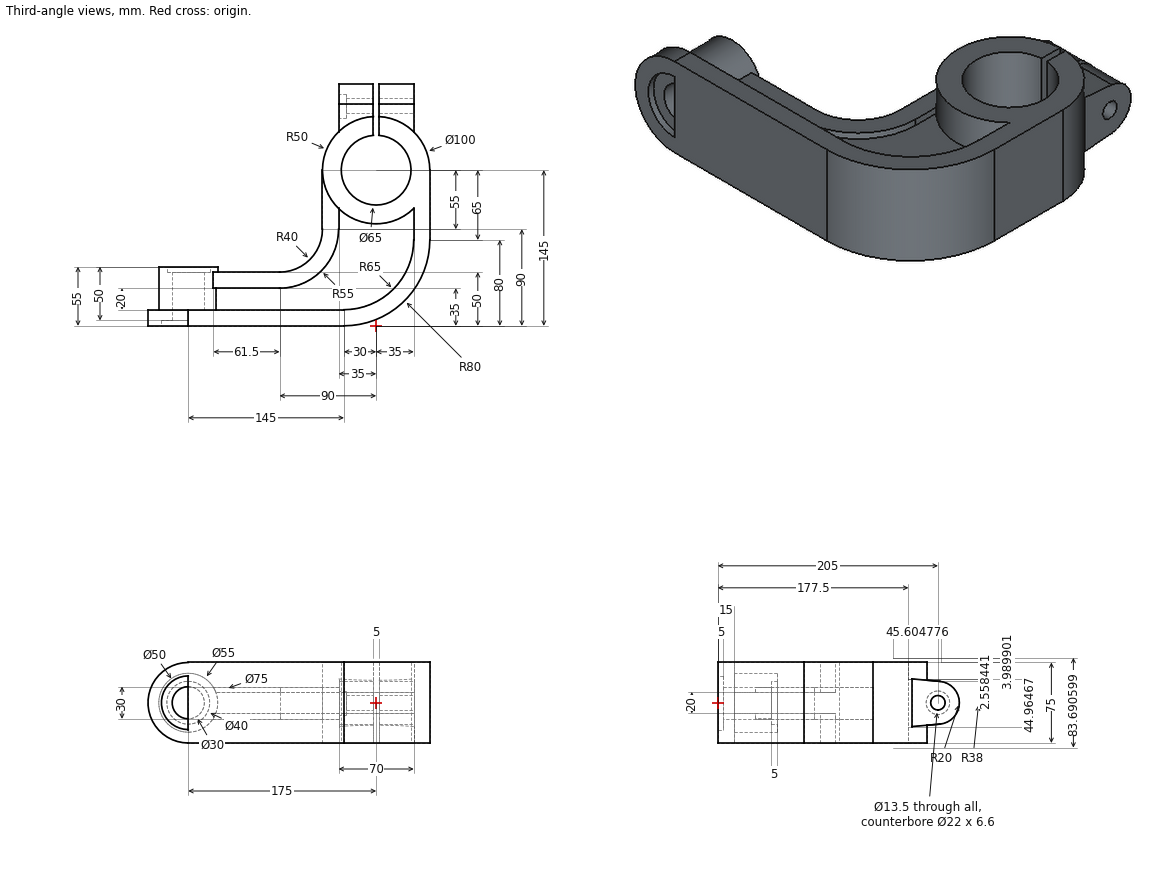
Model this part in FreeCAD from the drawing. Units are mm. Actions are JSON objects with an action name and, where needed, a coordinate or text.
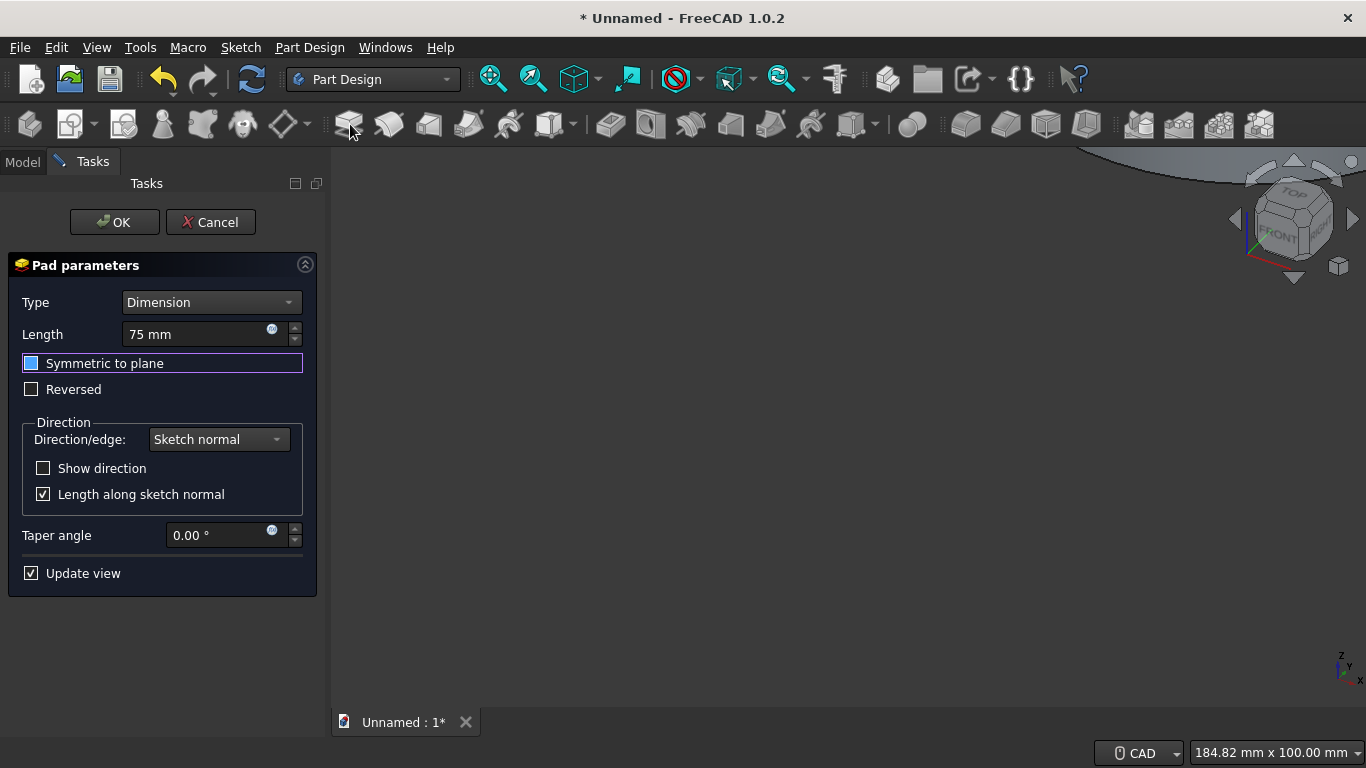
{"action": "left_click", "coordinate": [30, 363]}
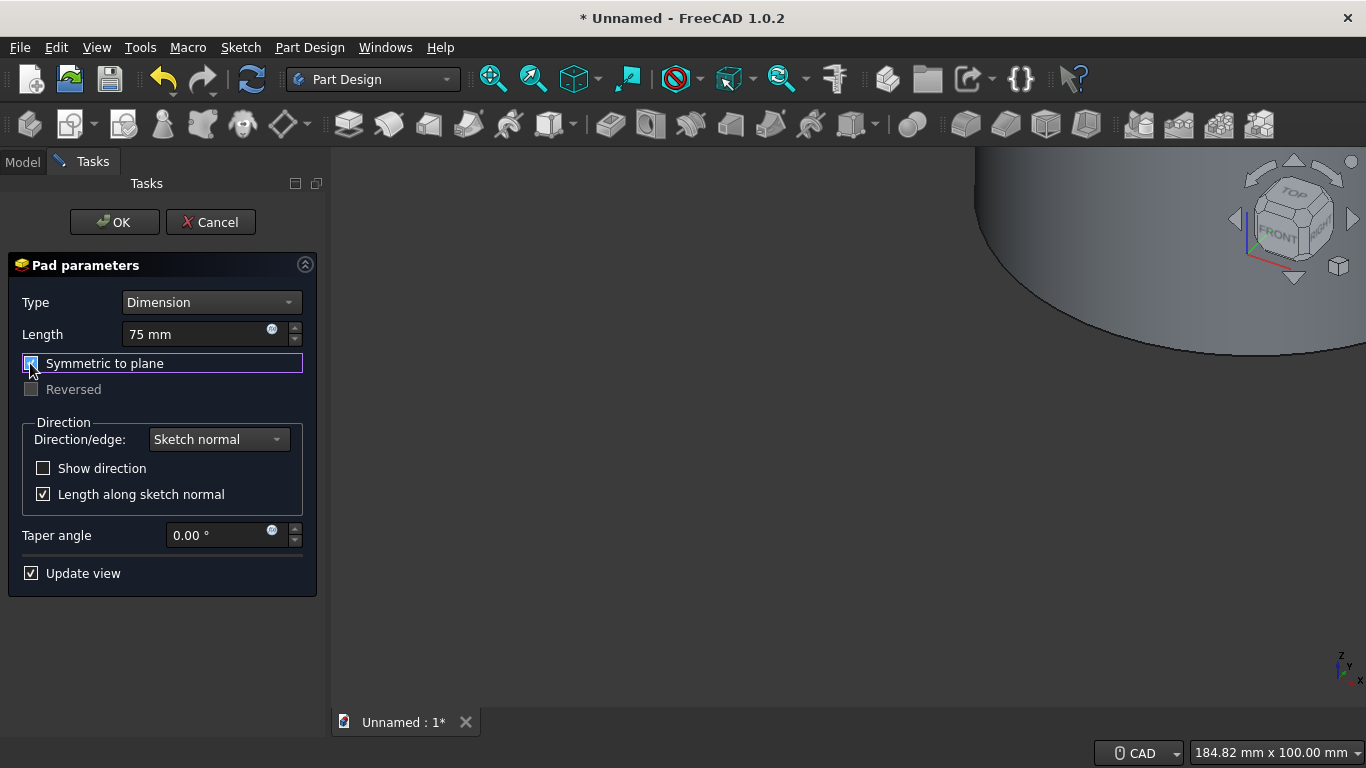
{"action": "left_click", "coordinate": [115, 222]}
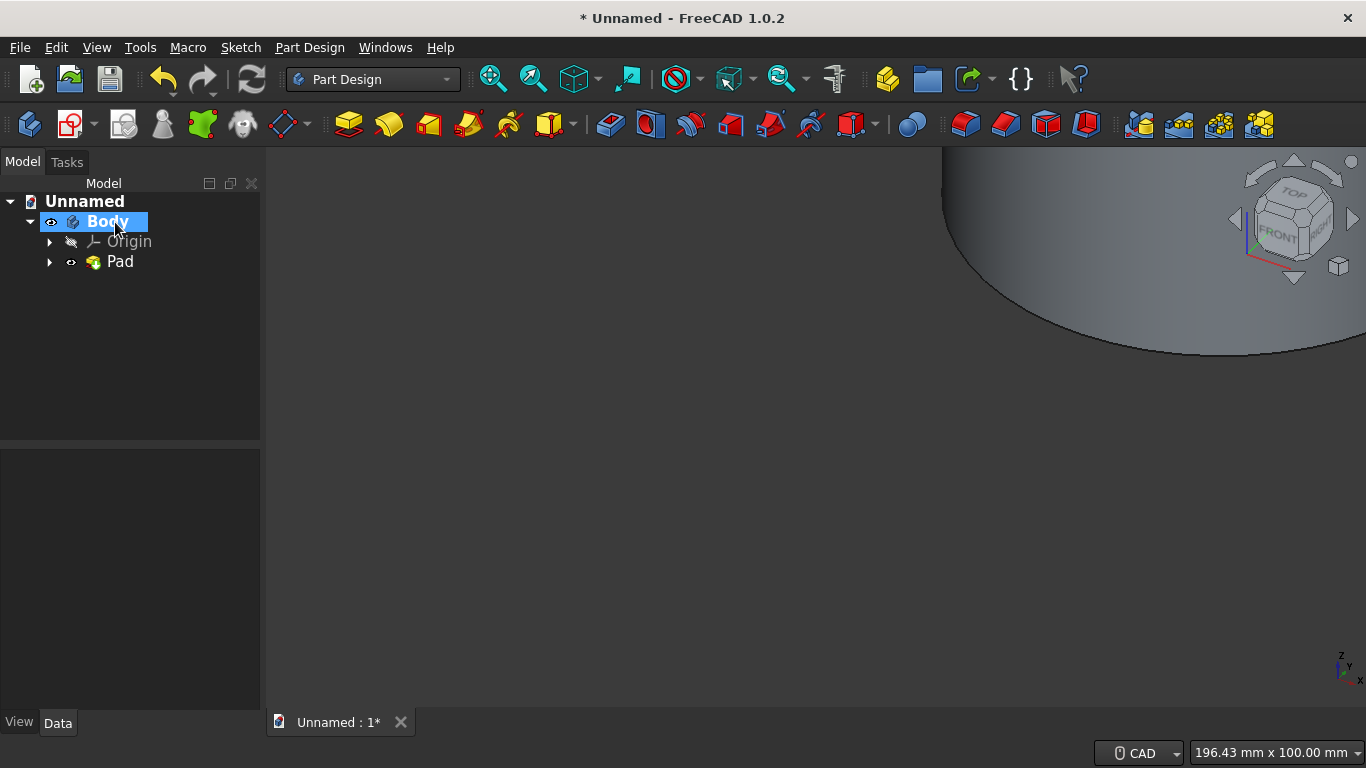
{"action": "left_click", "coordinate": [494, 80]}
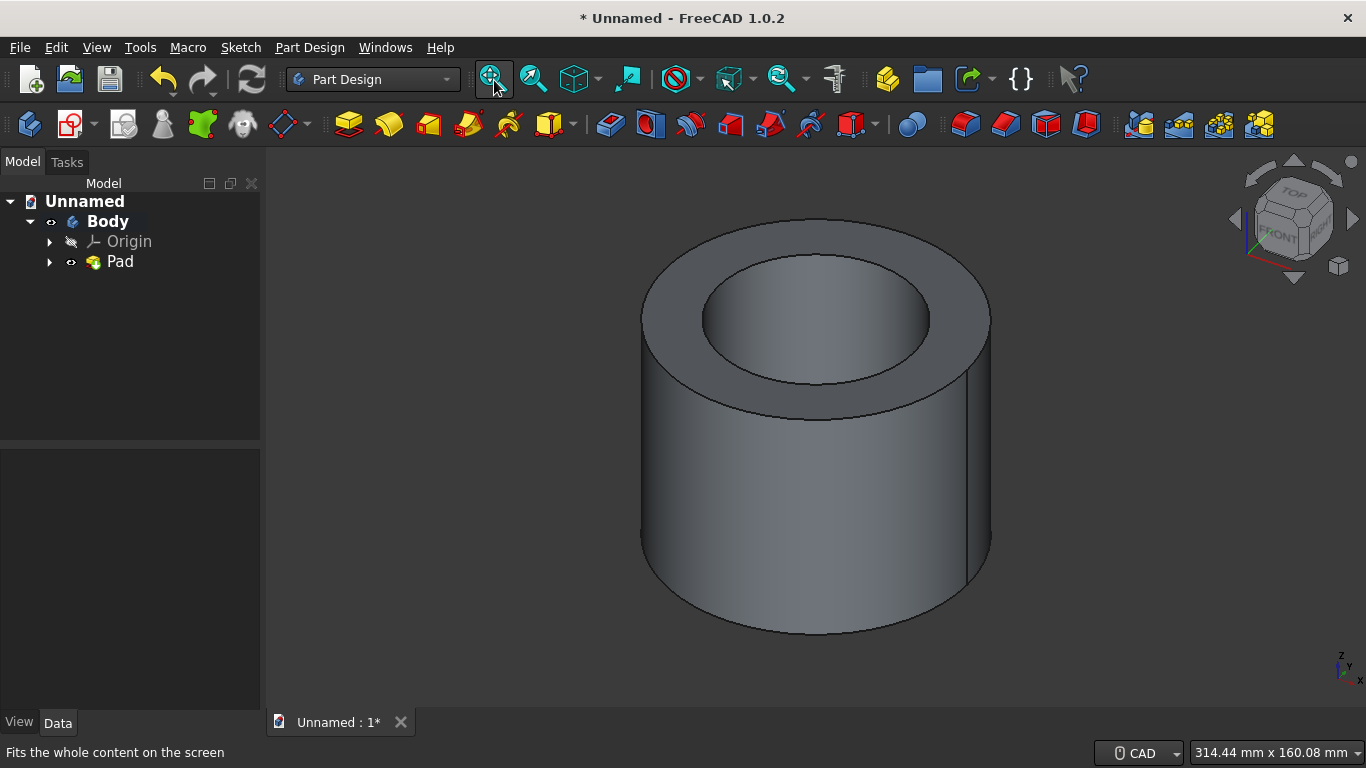
{"action": "left_click", "coordinate": [30, 124]}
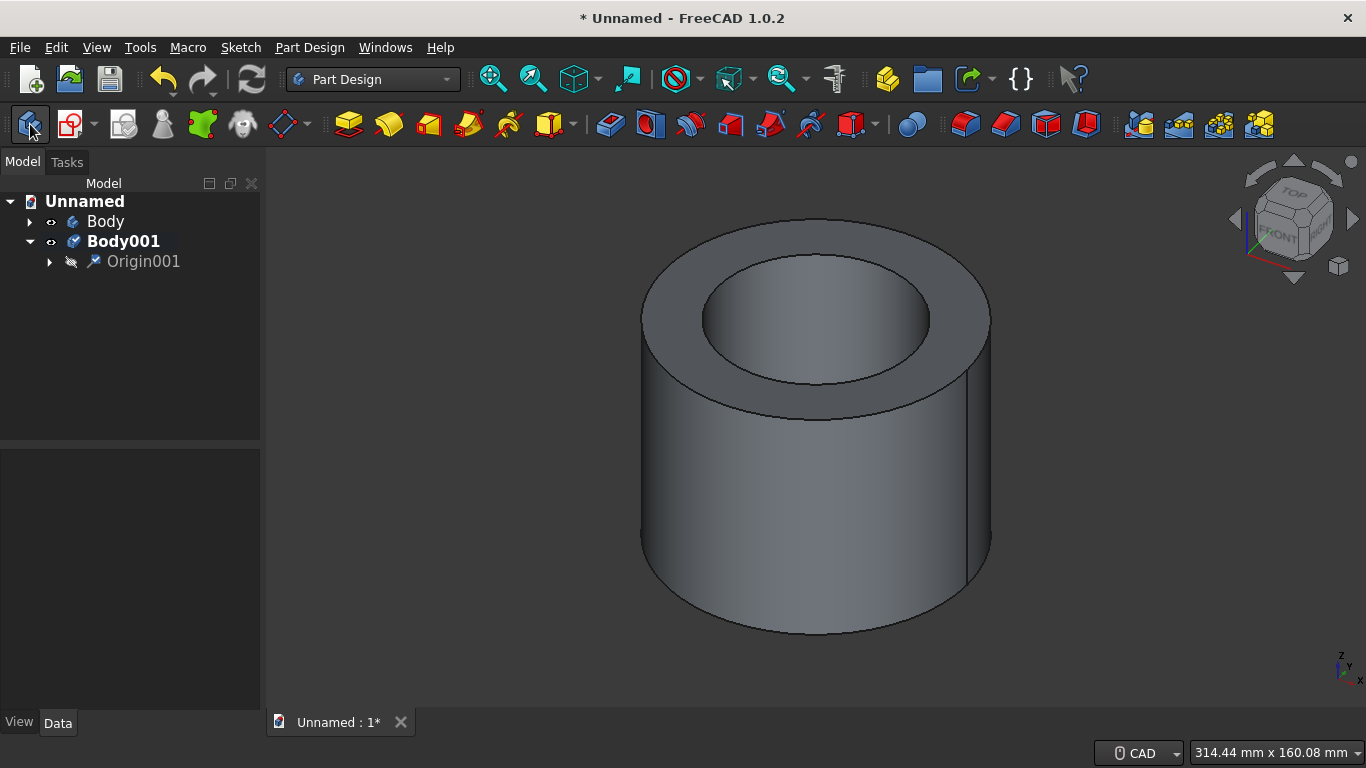
{"action": "left_click", "coordinate": [306, 667]}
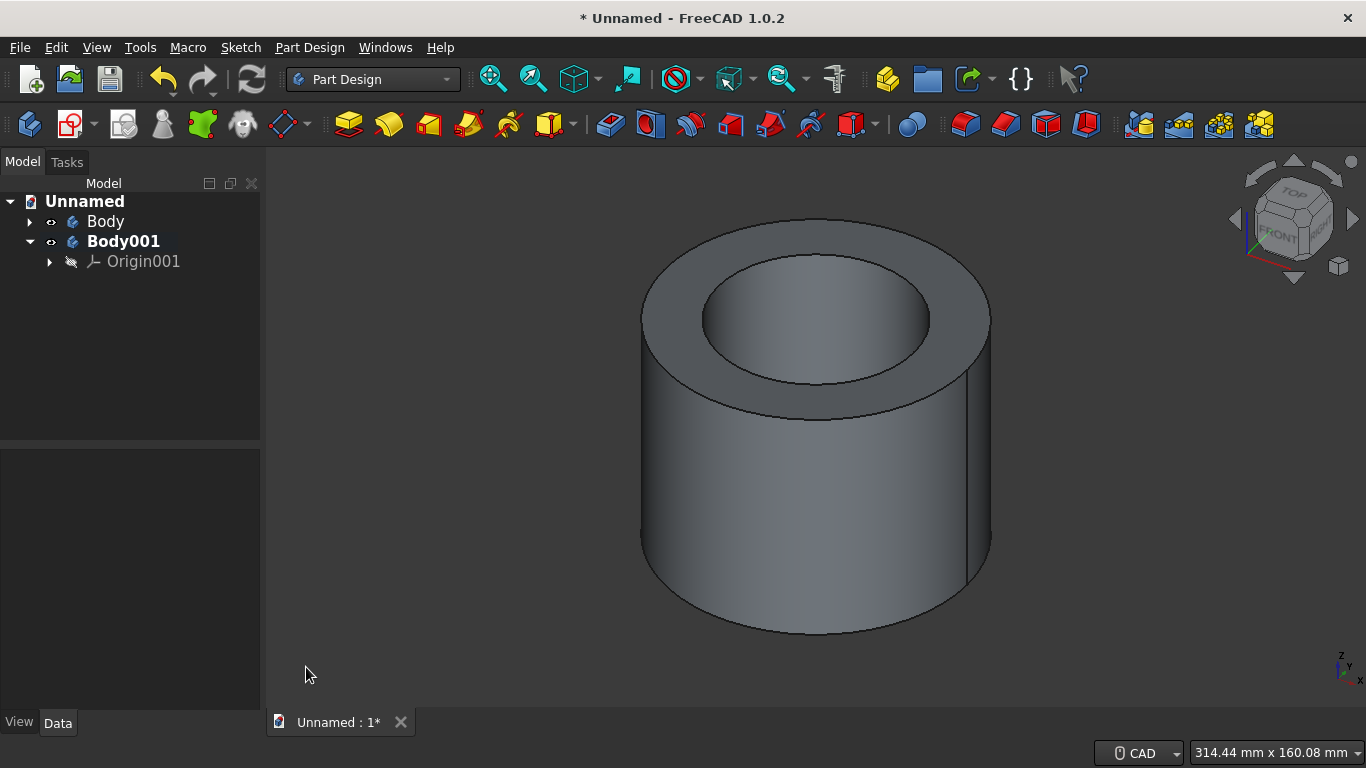
{"action": "left_click", "coordinate": [70, 124]}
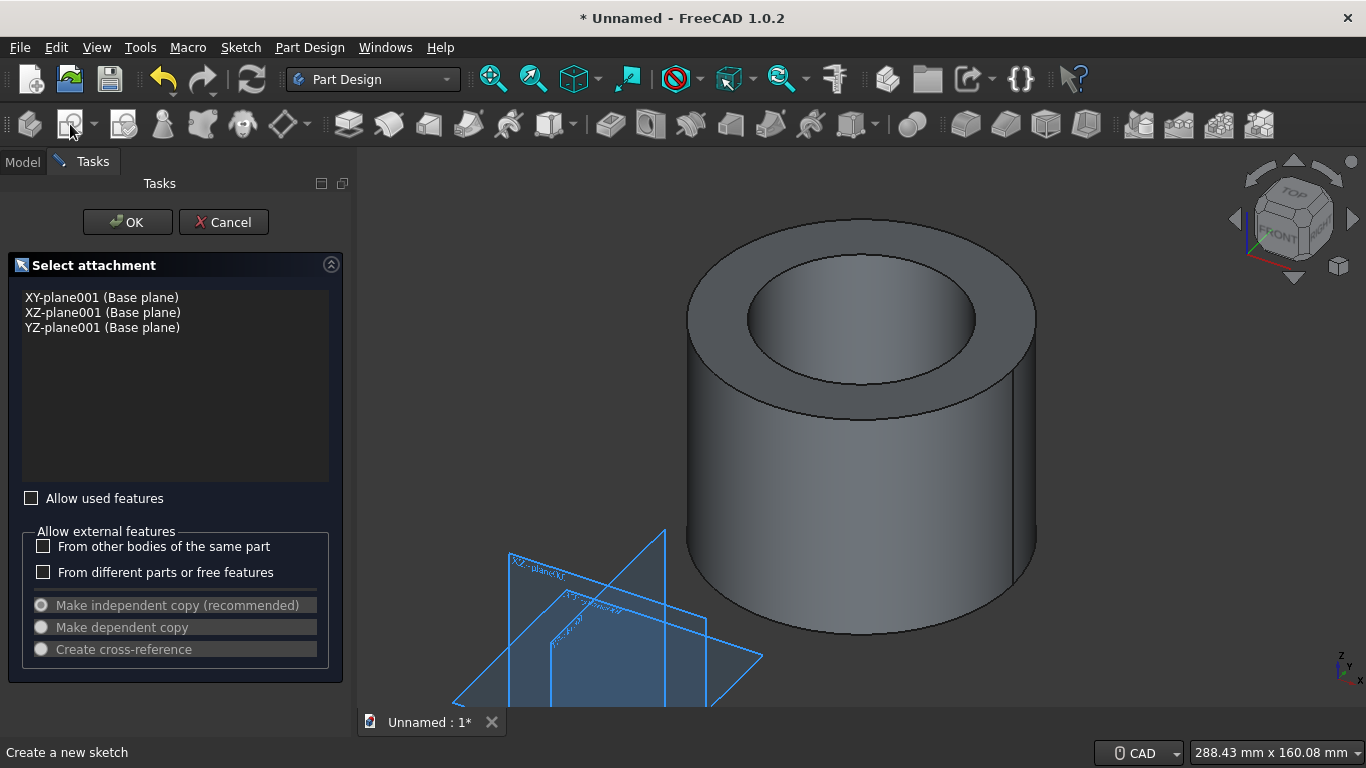
{"action": "left_click", "coordinate": [82, 312]}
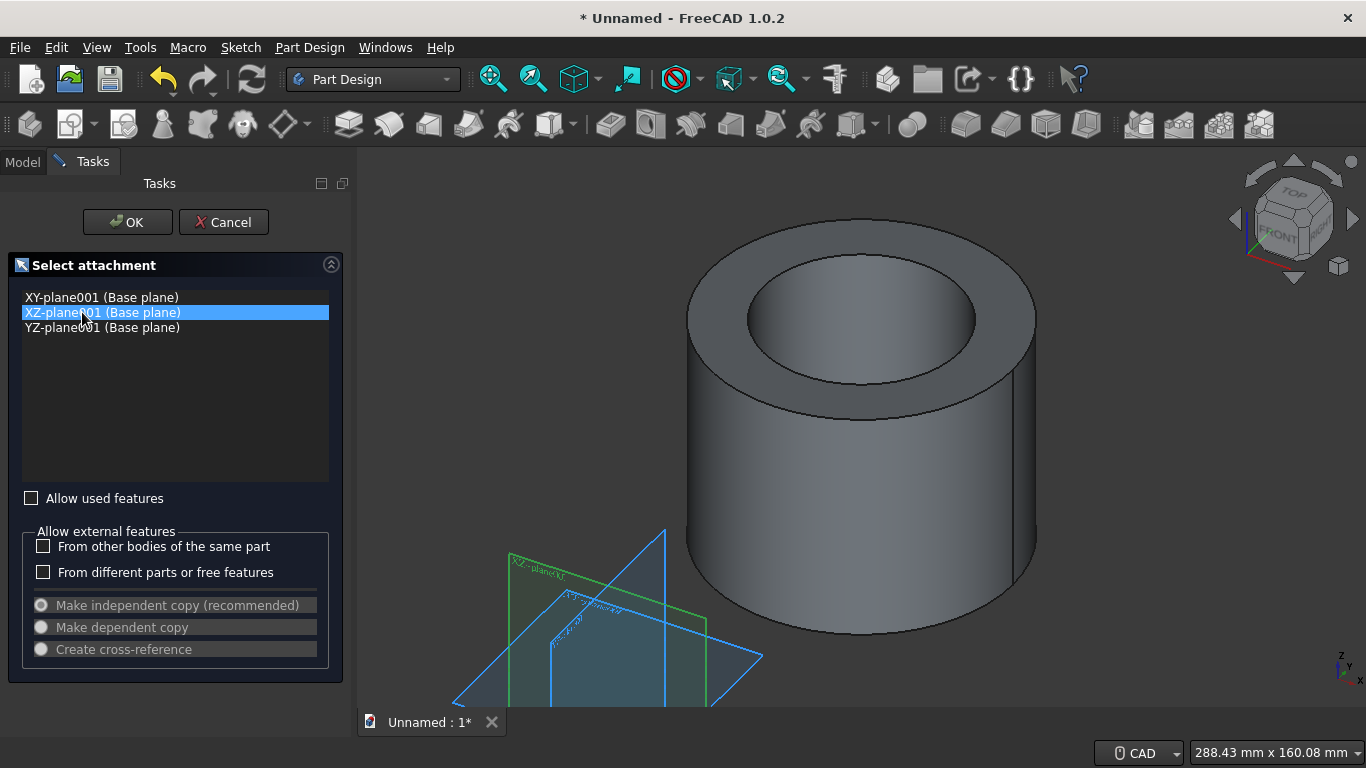
{"action": "left_click", "coordinate": [128, 222]}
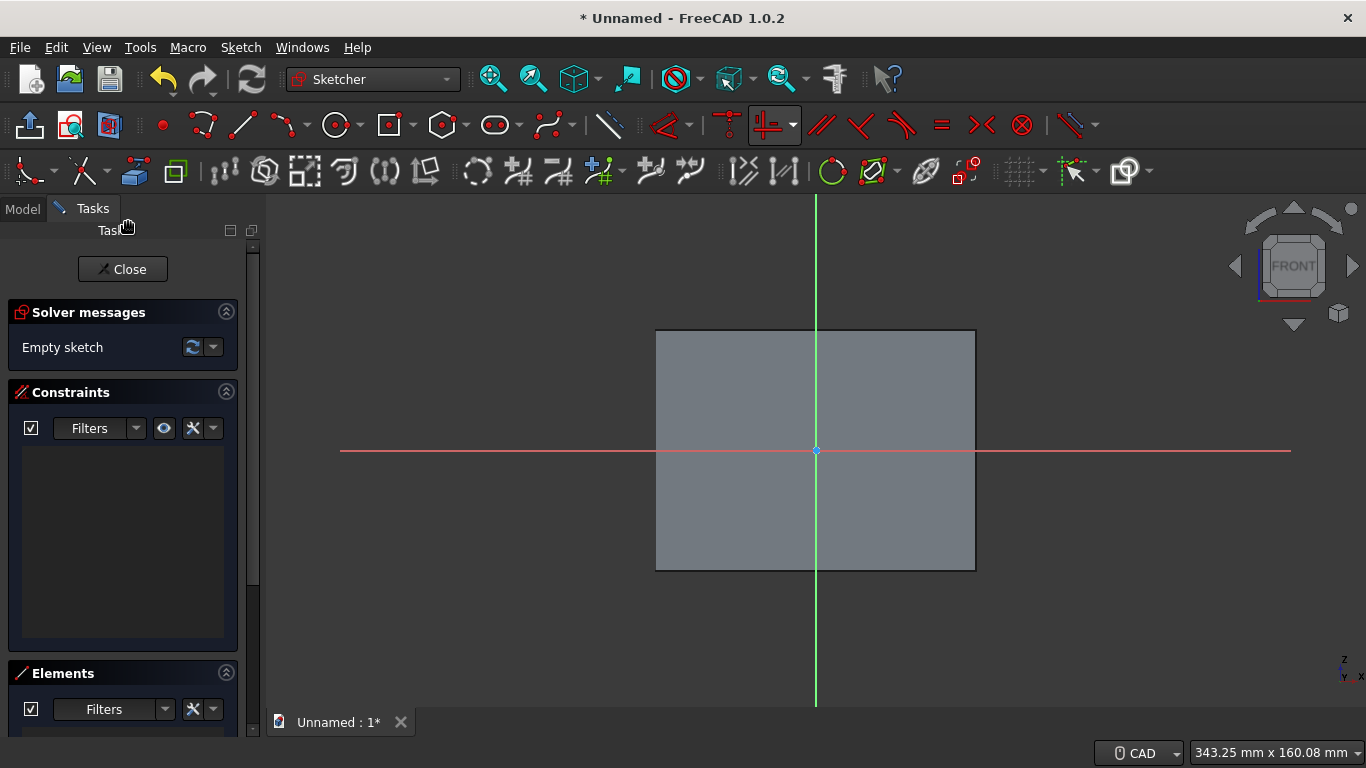
{"action": "scroll", "coordinate": [1201, 450], "scroll_direction": "down", "scroll_amount": 1}